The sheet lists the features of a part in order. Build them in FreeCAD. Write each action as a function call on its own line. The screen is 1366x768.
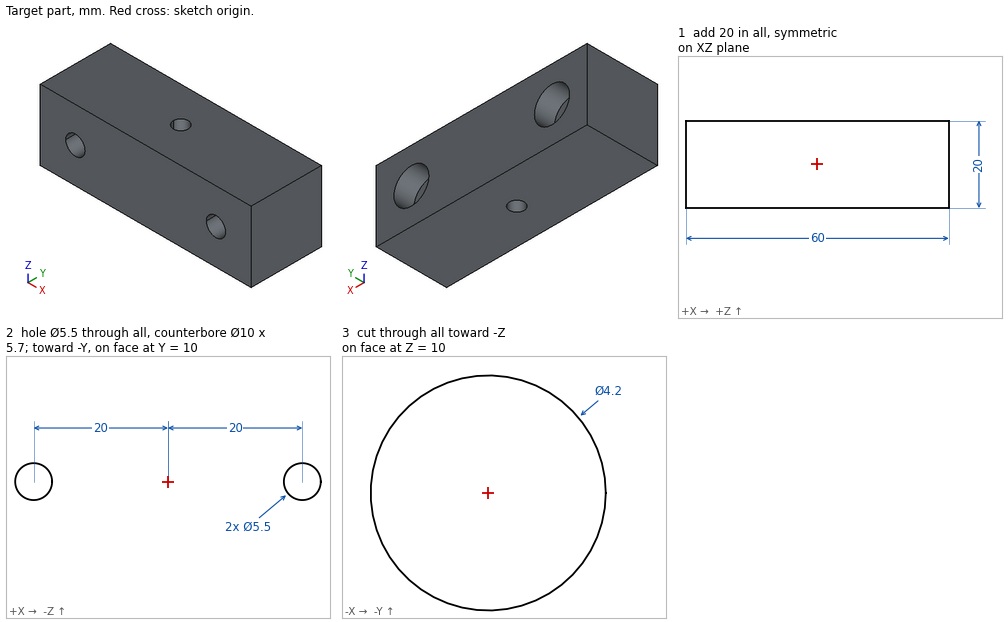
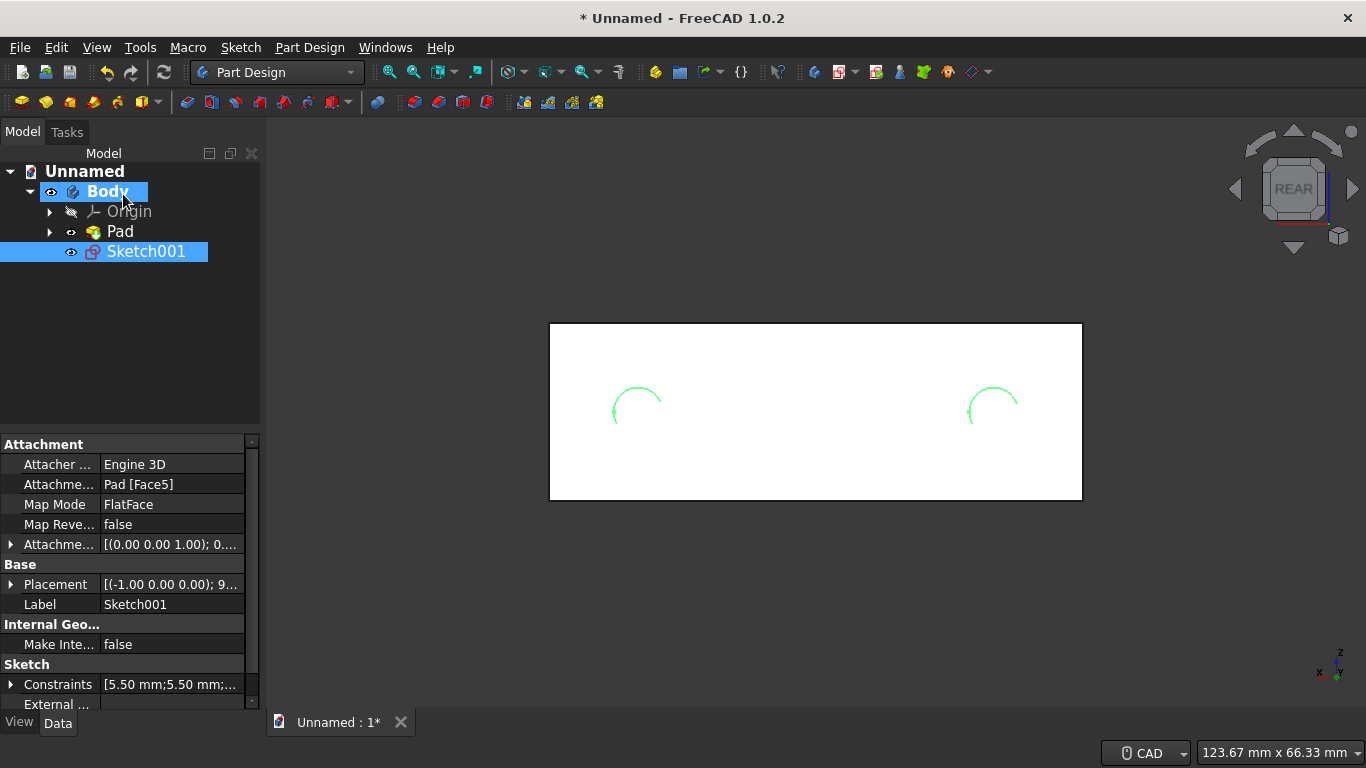
click(212, 102)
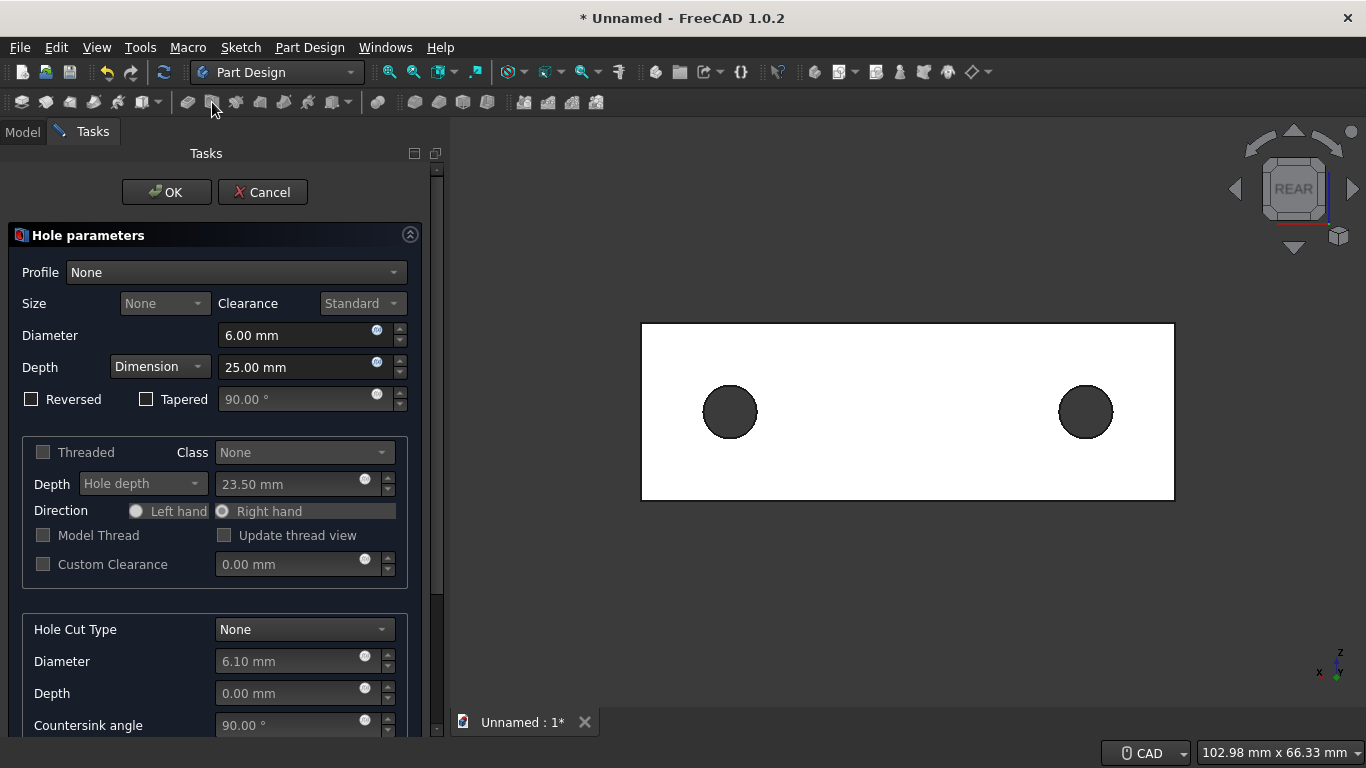
triple_click(305, 335)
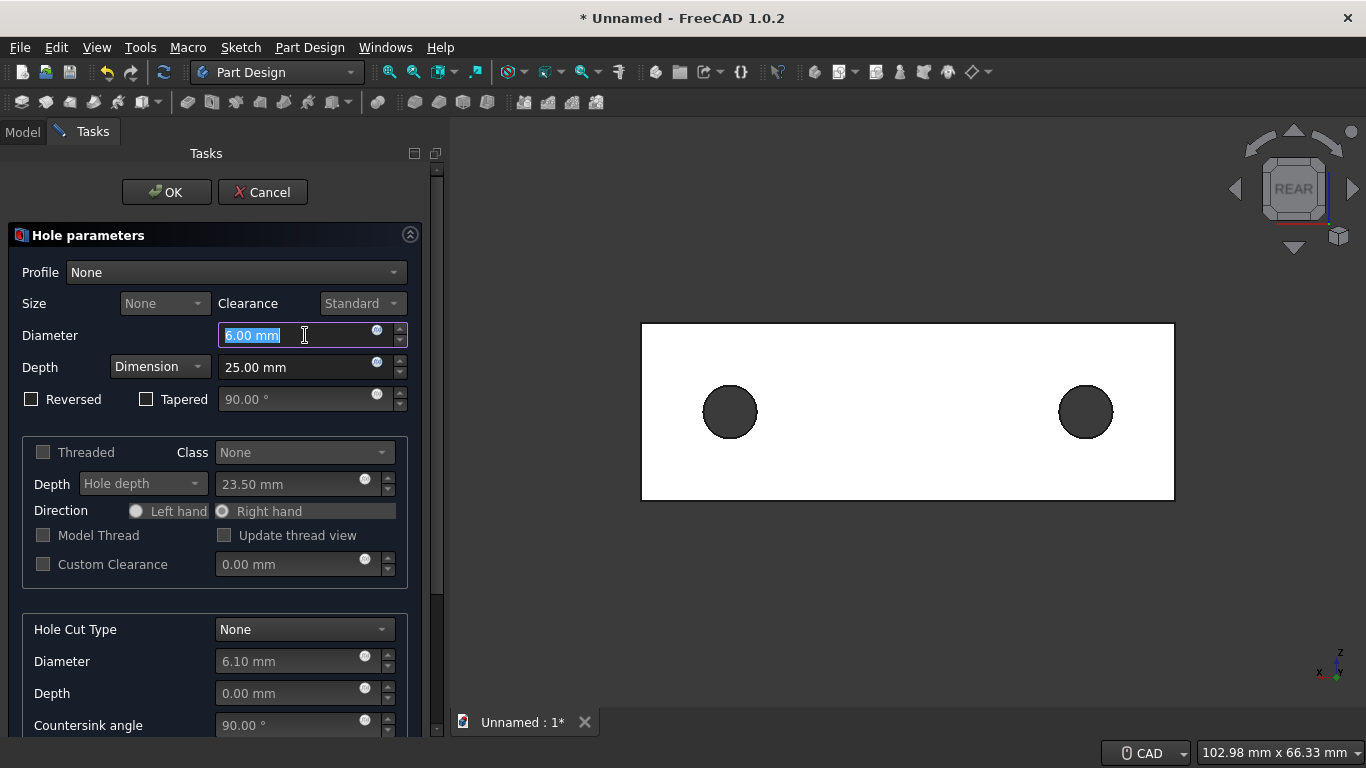
text(5.5)
key(Tab)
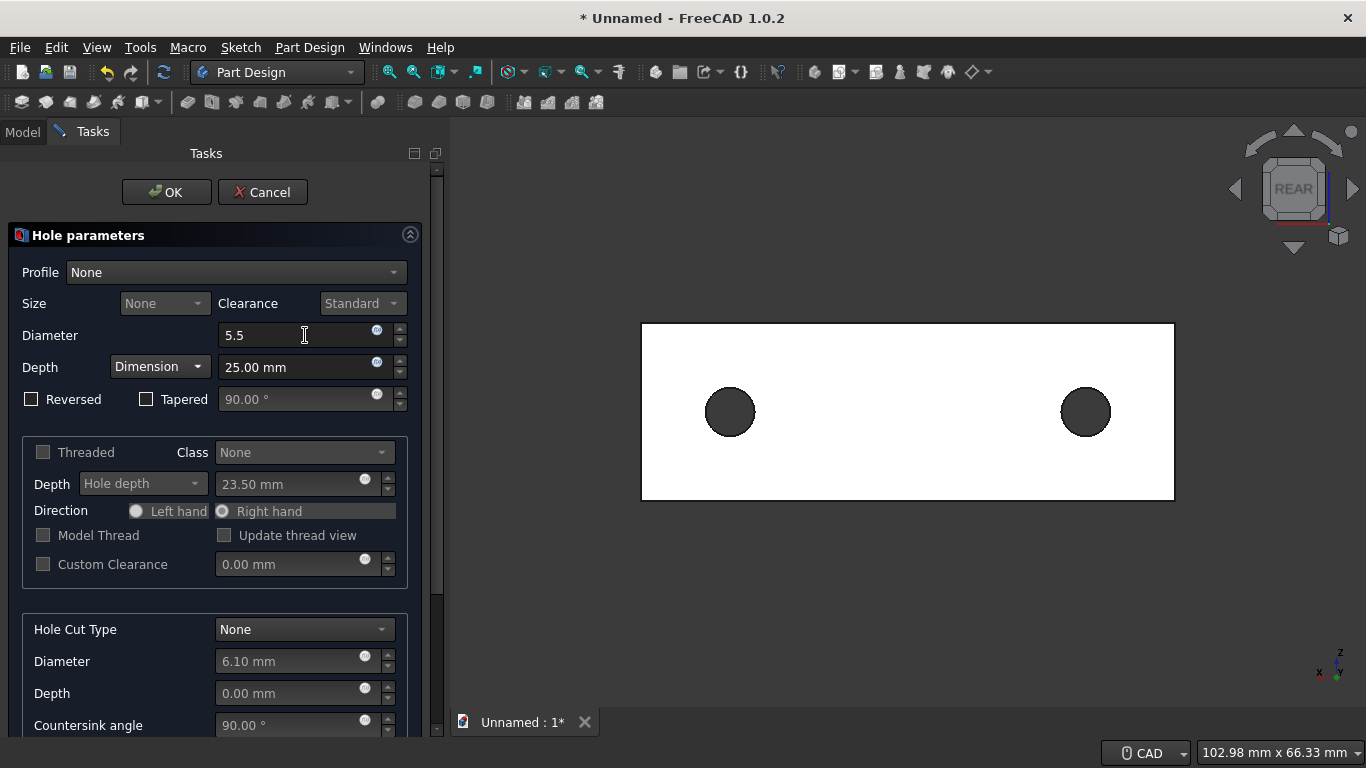
click(161, 366)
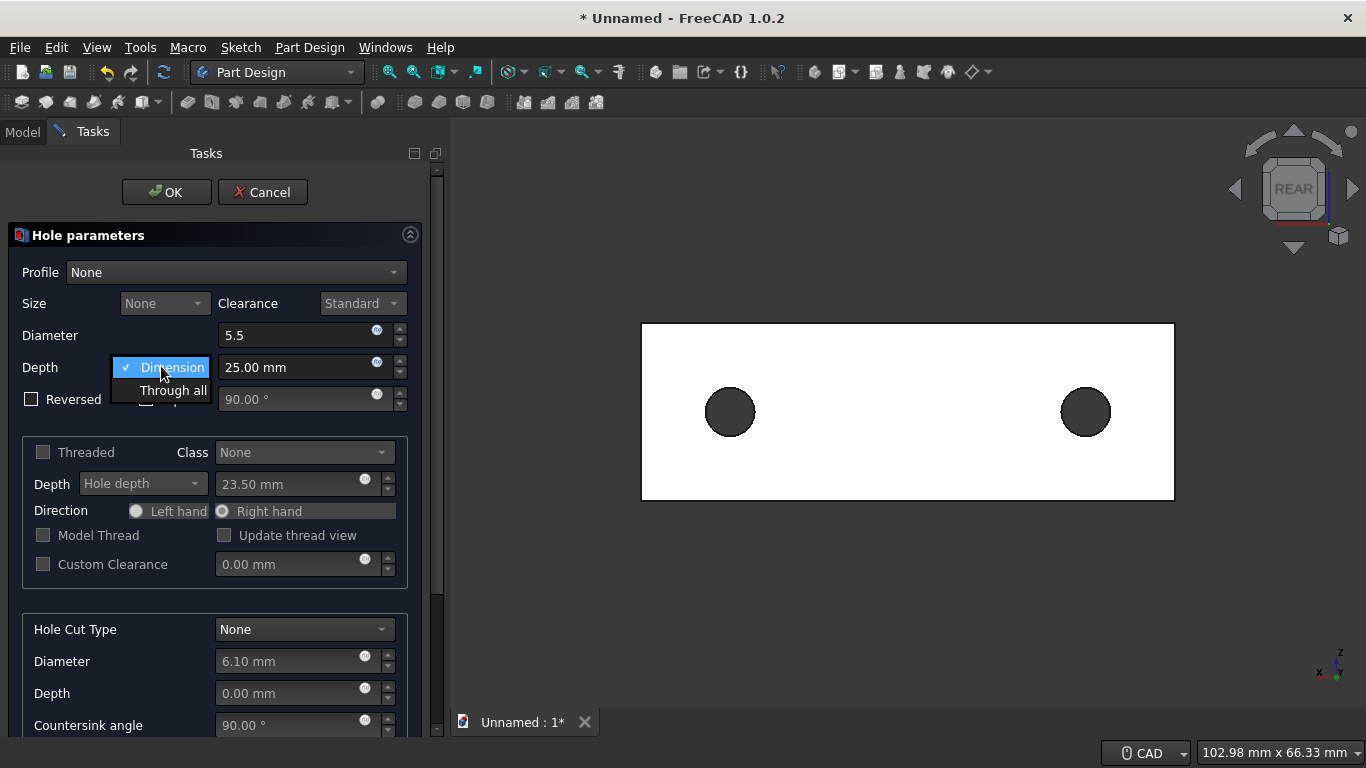
click(160, 390)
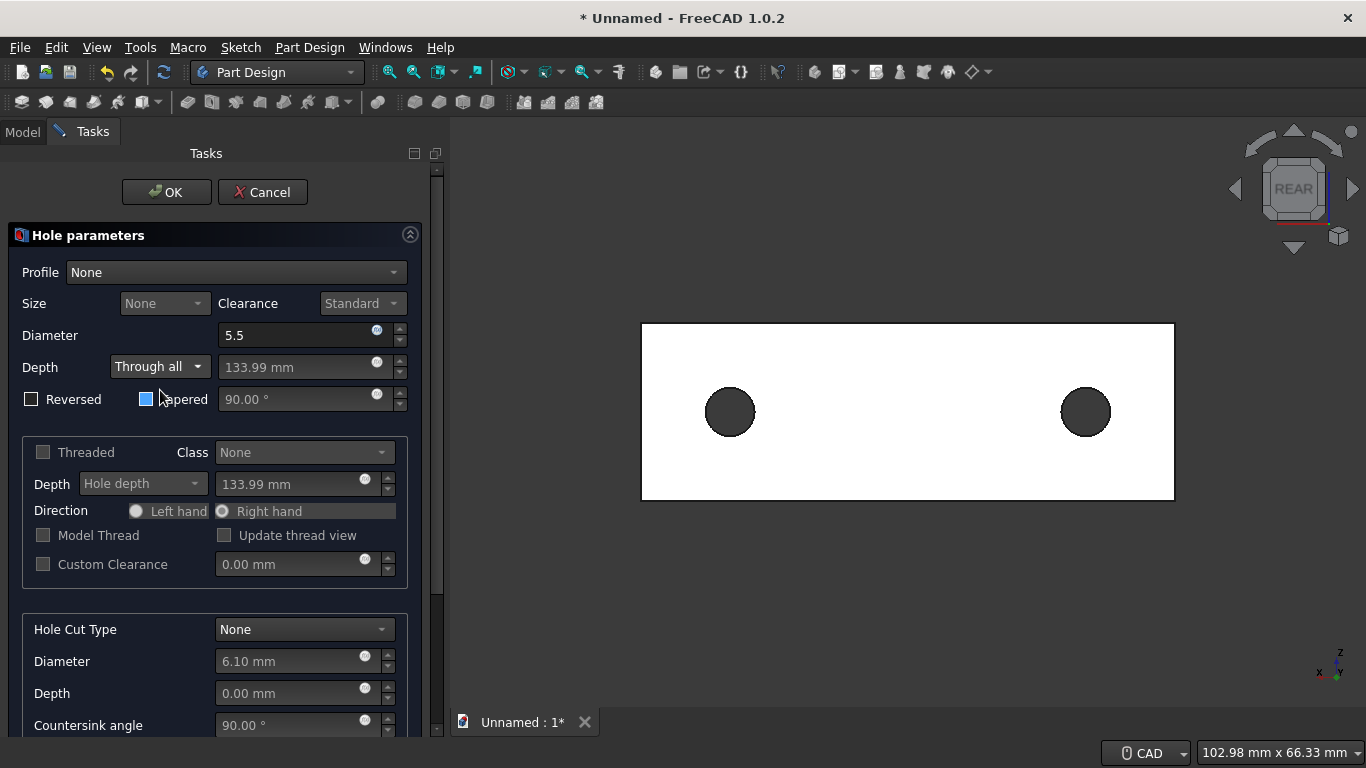
click(306, 630)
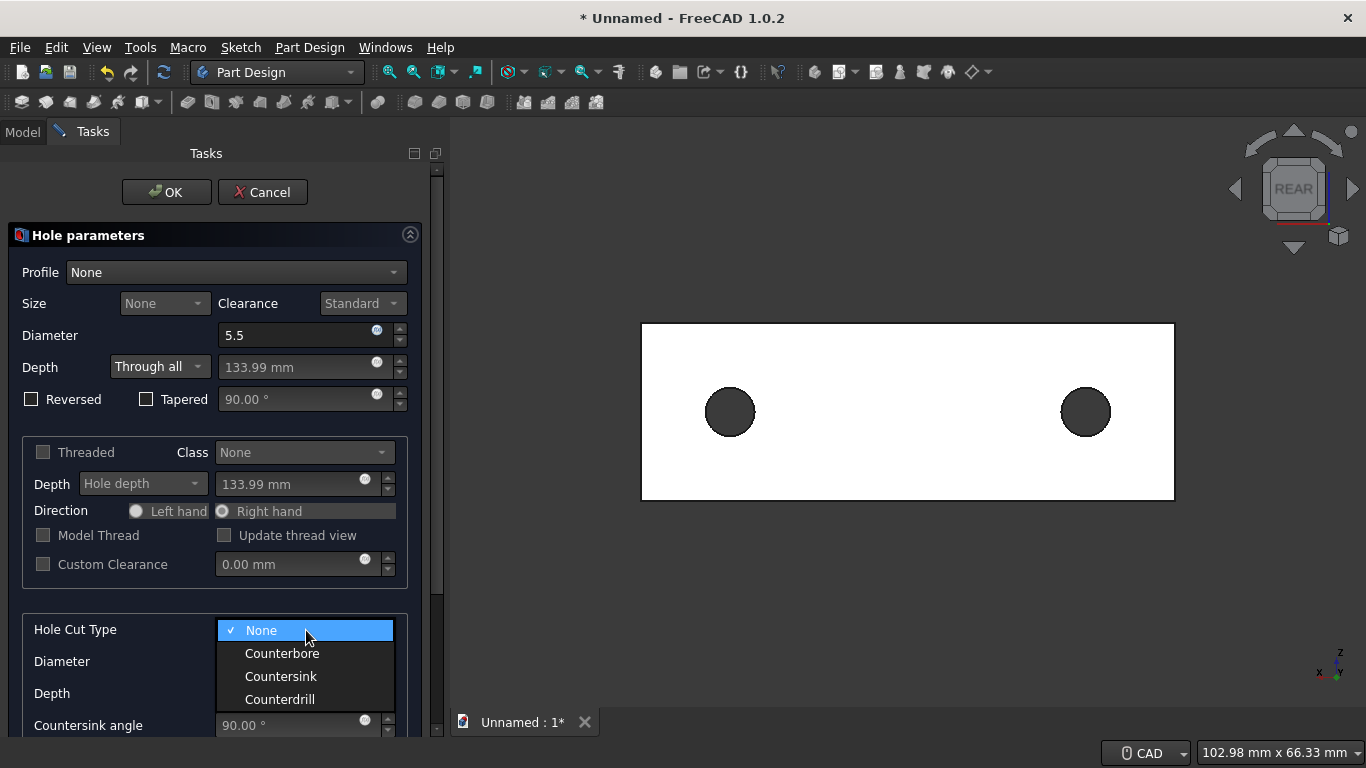
click(304, 654)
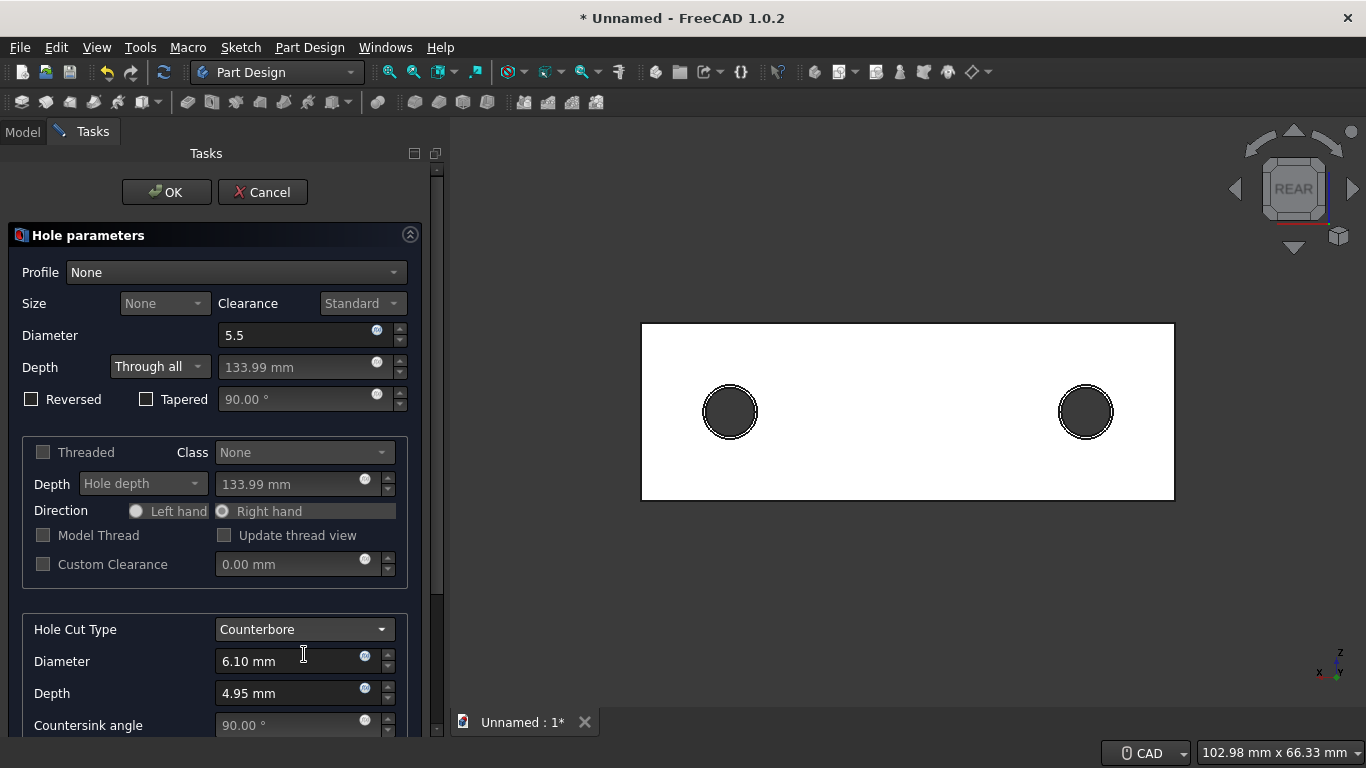
triple_click(298, 661)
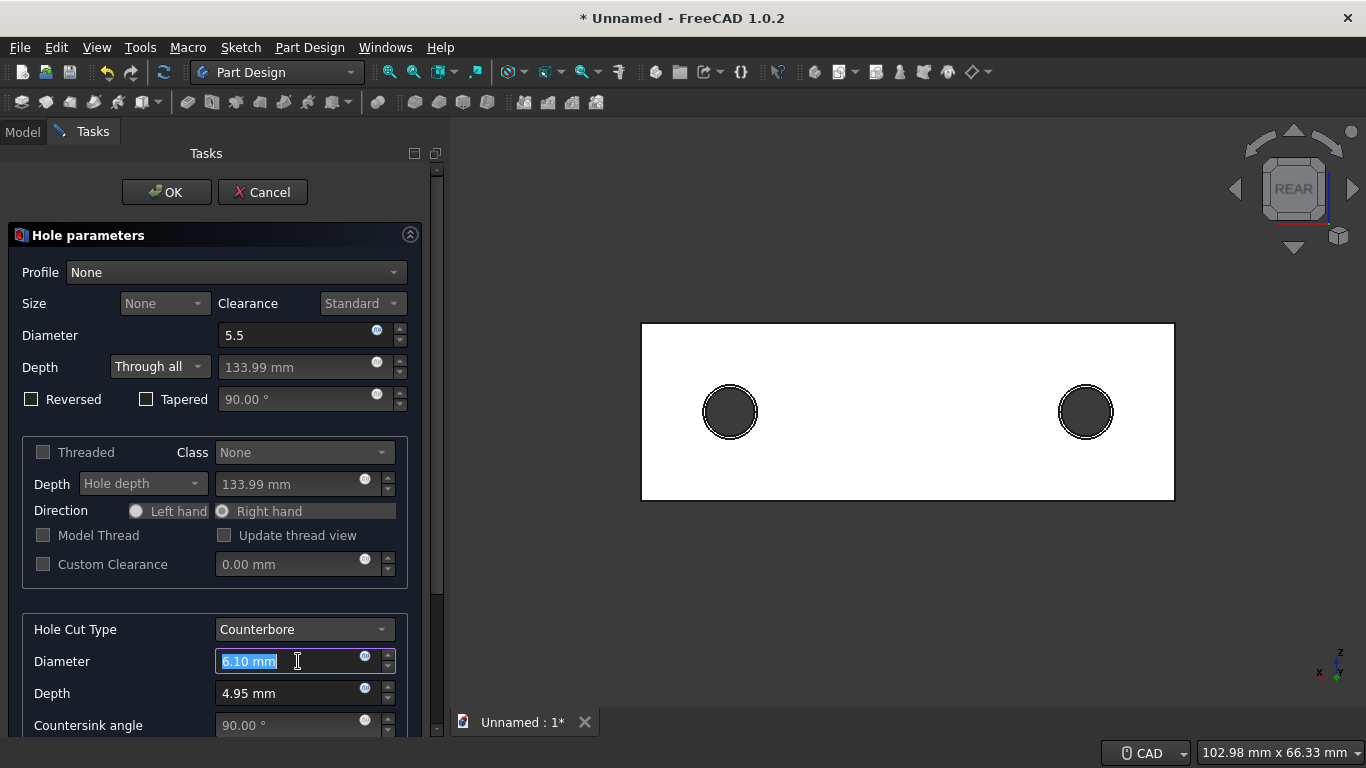
text(10)
key(Tab)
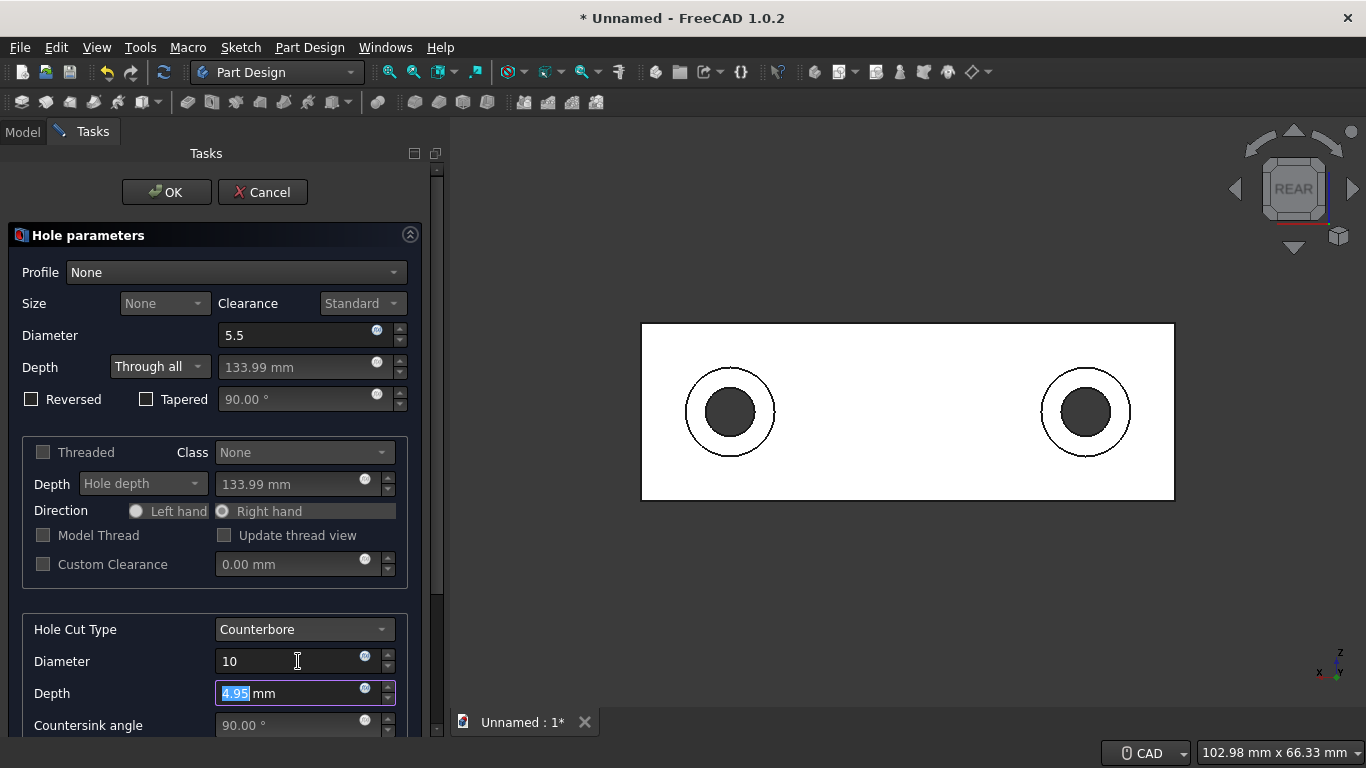
text(5.7)
key(Tab)